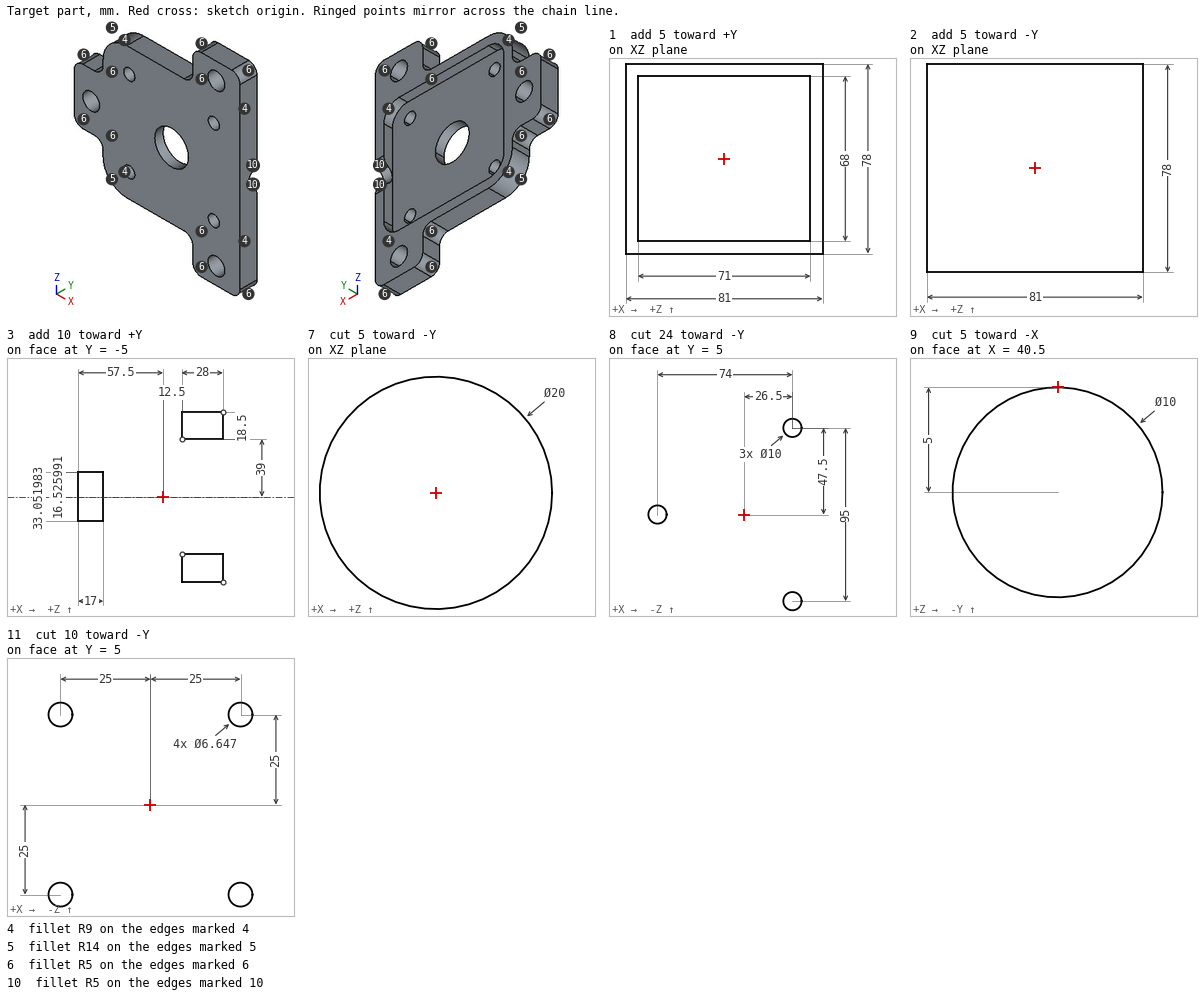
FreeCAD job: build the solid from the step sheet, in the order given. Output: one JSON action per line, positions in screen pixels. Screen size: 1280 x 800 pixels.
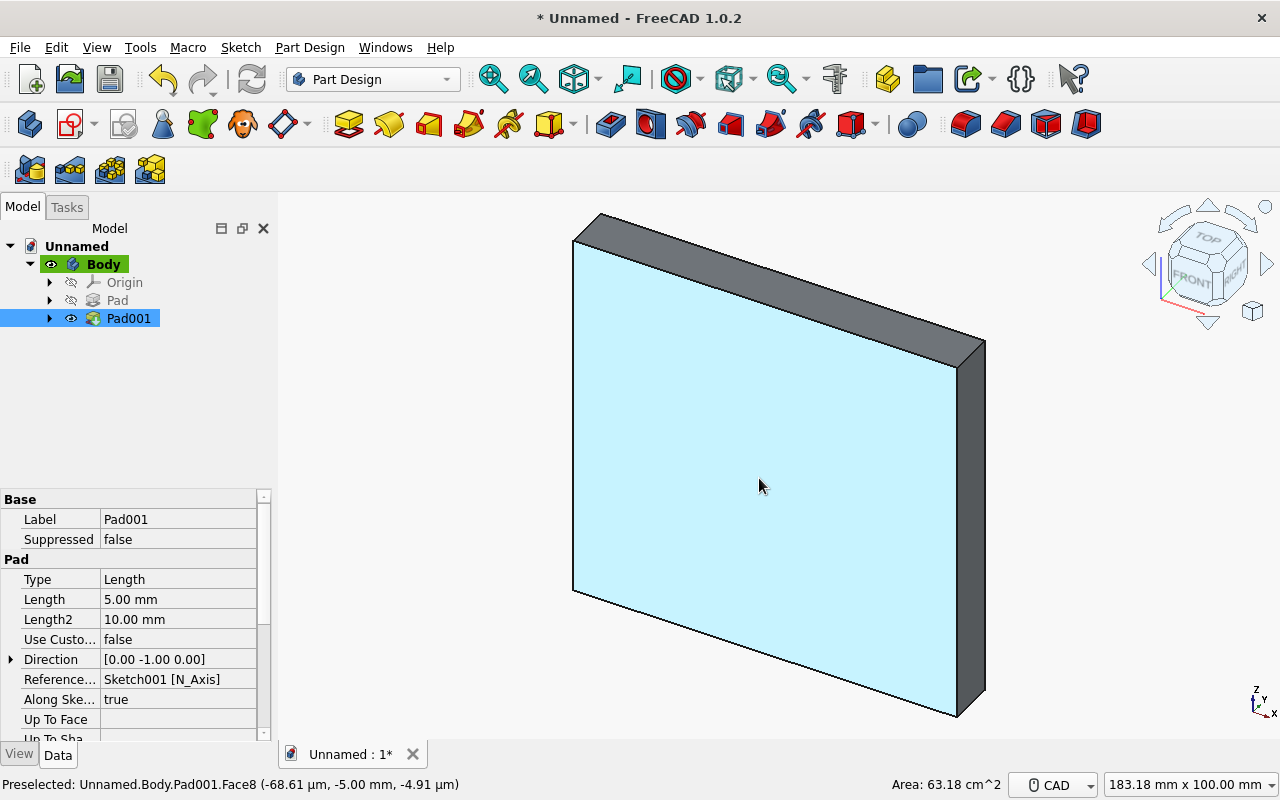
{"action": "left_click", "coordinate": [70, 124]}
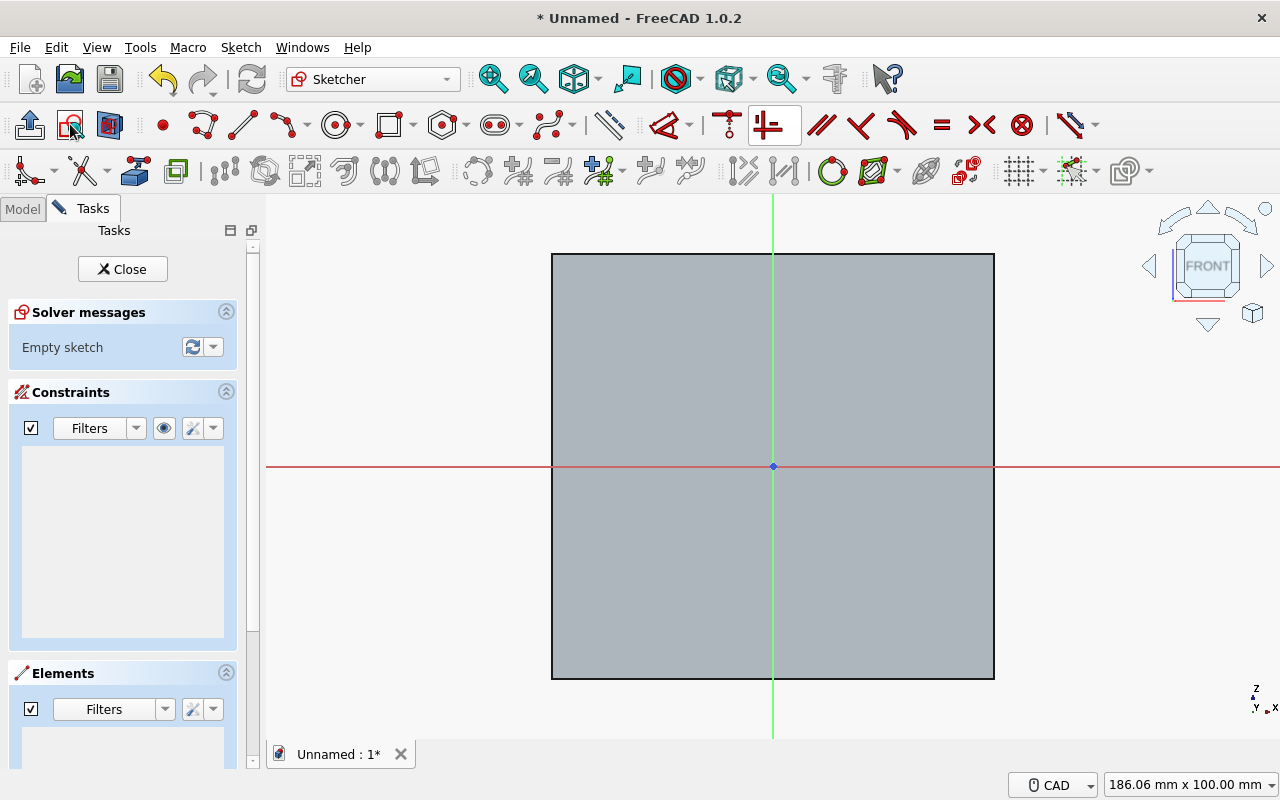
{"action": "scroll", "coordinate": [678, 466], "scroll_direction": "down", "scroll_amount": 3}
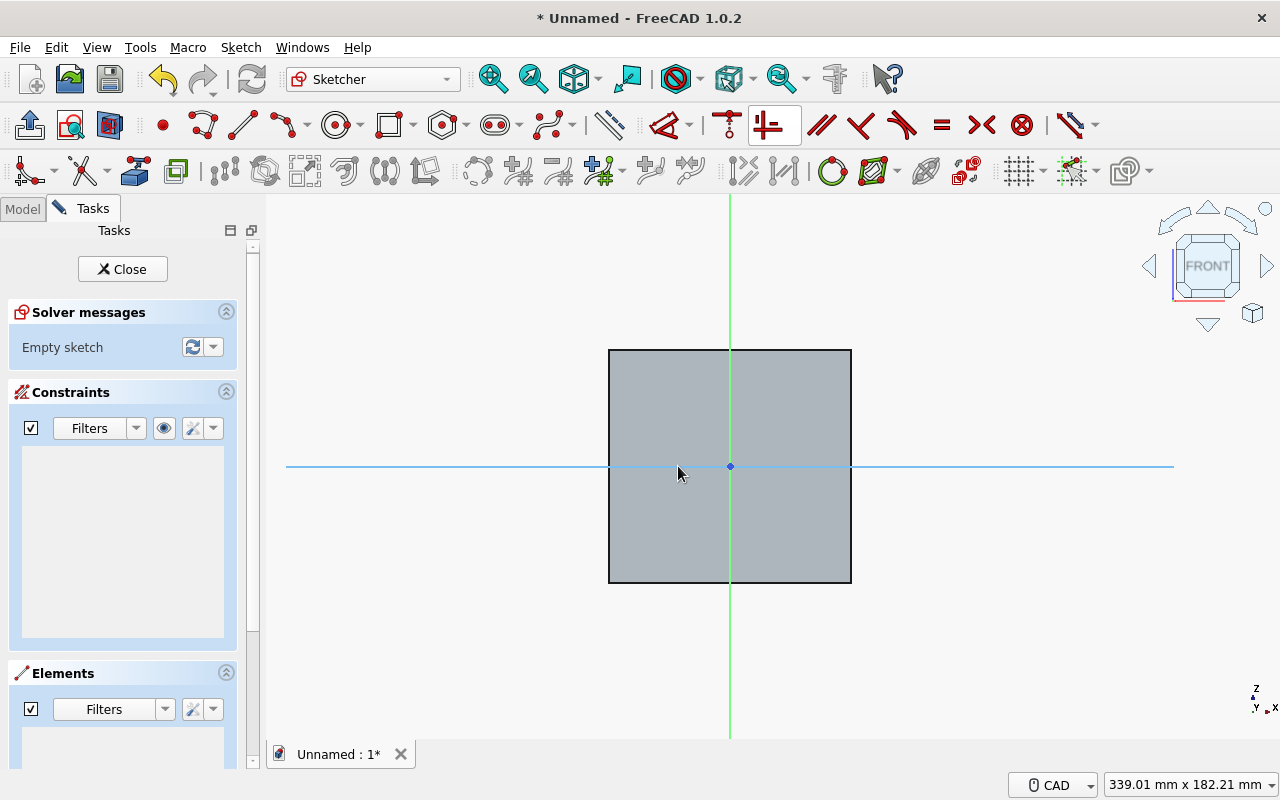
{"action": "left_click", "coordinate": [390, 126]}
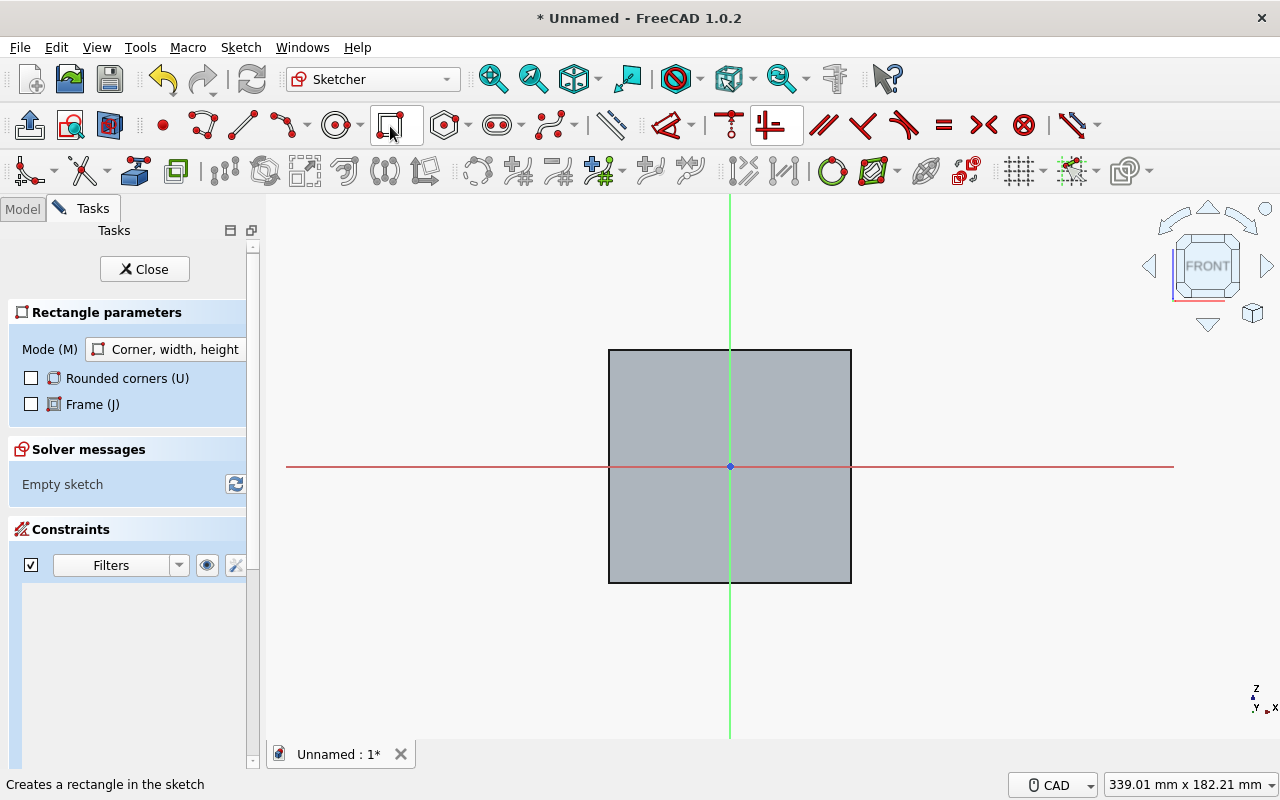
{"action": "left_click", "coordinate": [558, 417]}
{"action": "left_click", "coordinate": [609, 516]}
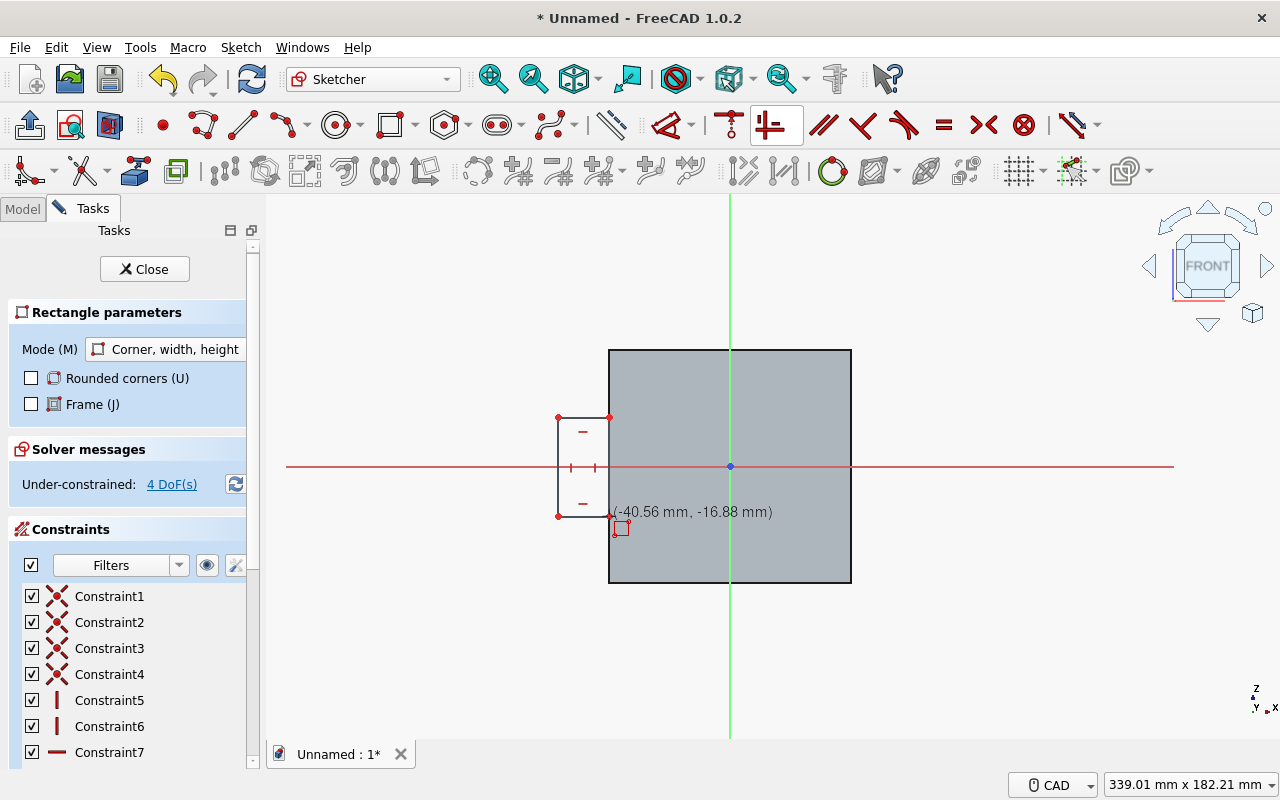
{"action": "left_click", "coordinate": [768, 295]}
{"action": "left_click", "coordinate": [851, 350]}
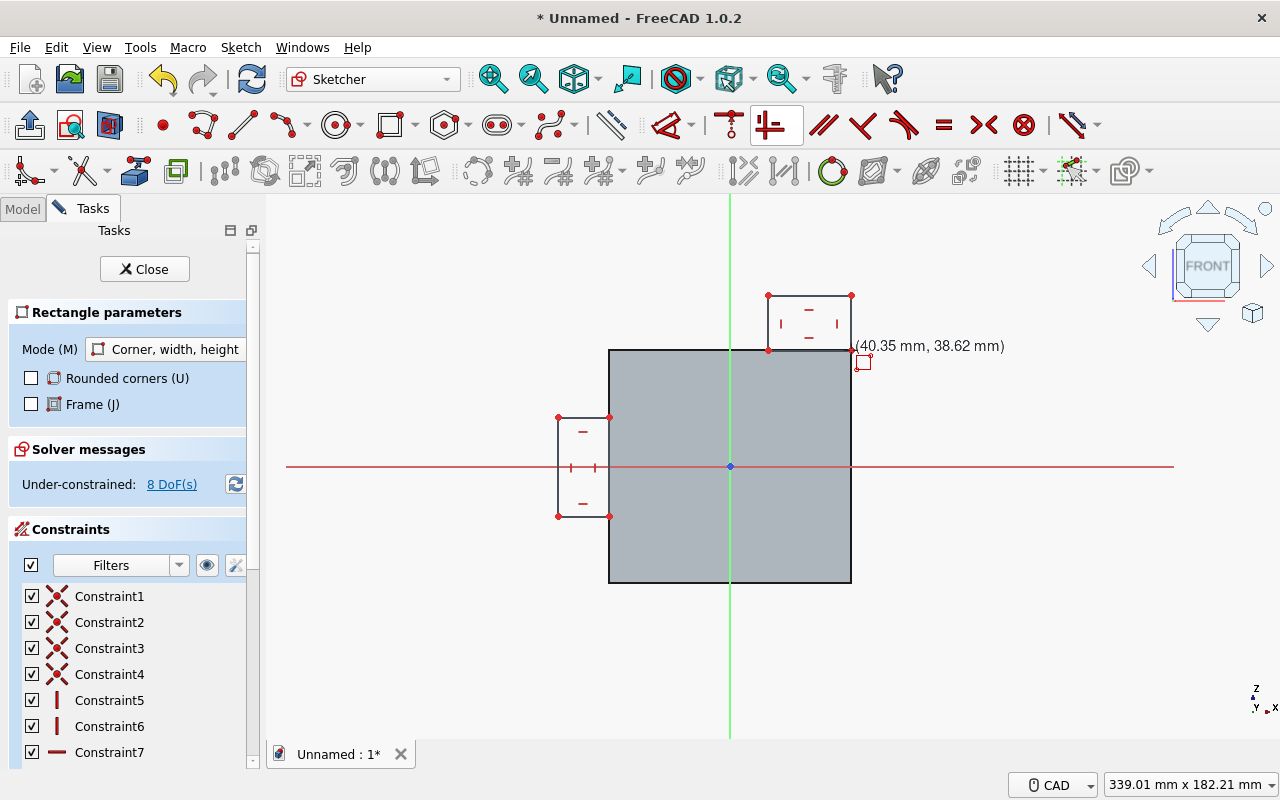
{"action": "left_click", "coordinate": [768, 583]}
{"action": "left_click", "coordinate": [851, 638]}
{"action": "key", "text": "Escape"}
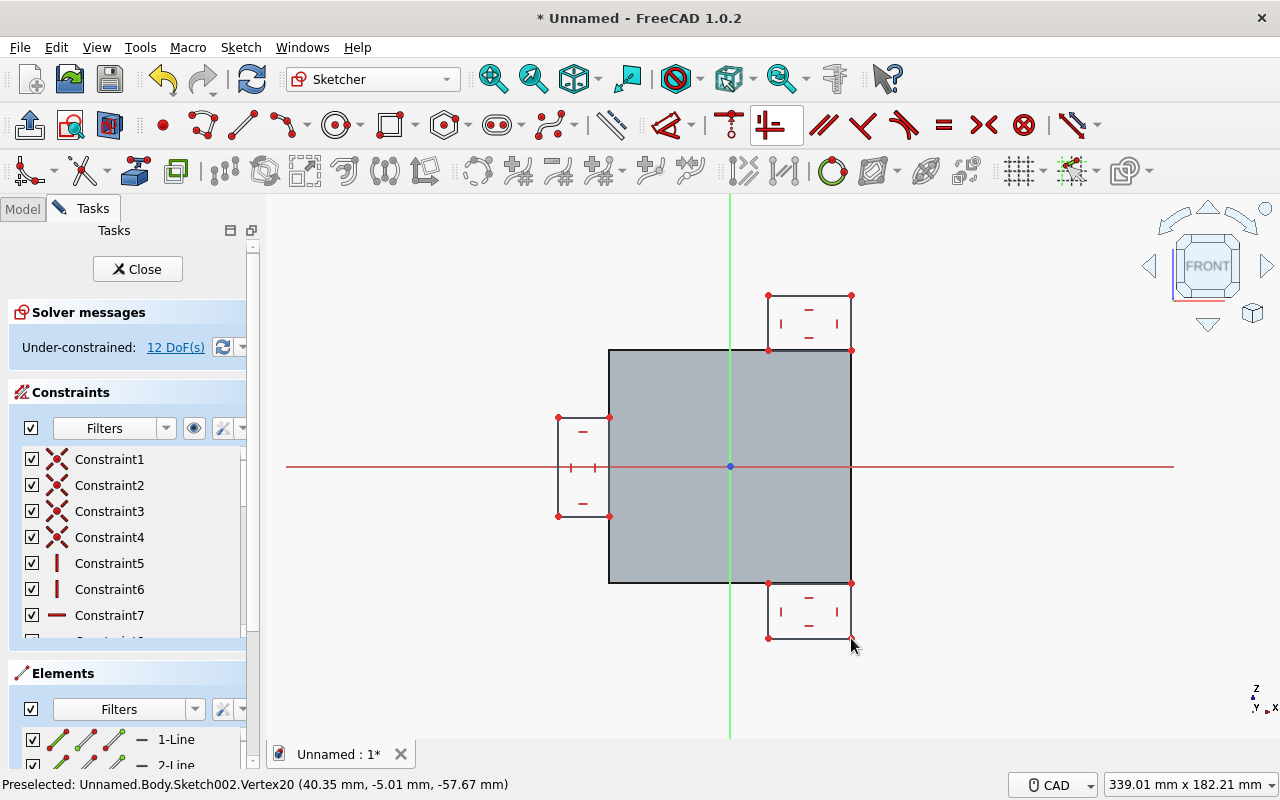
{"action": "left_click", "coordinate": [768, 351]}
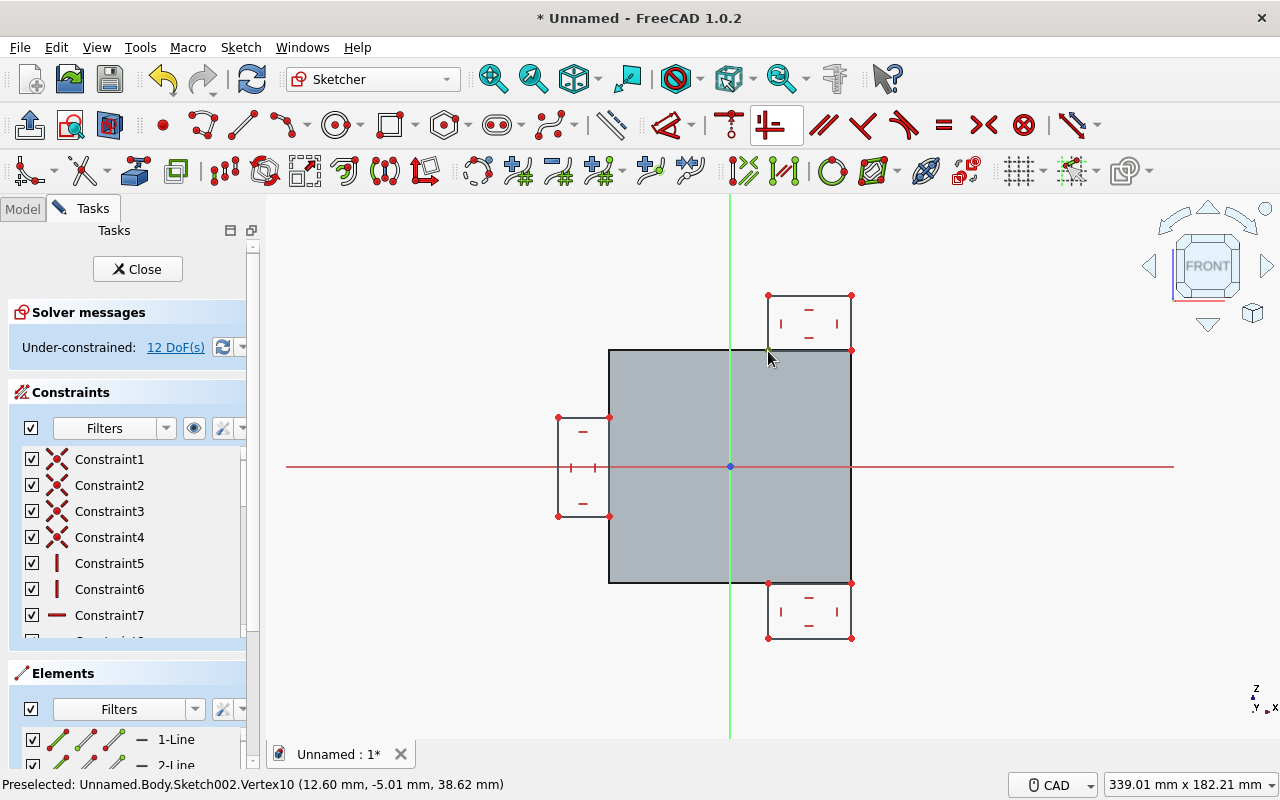
{"action": "left_click", "coordinate": [768, 584]}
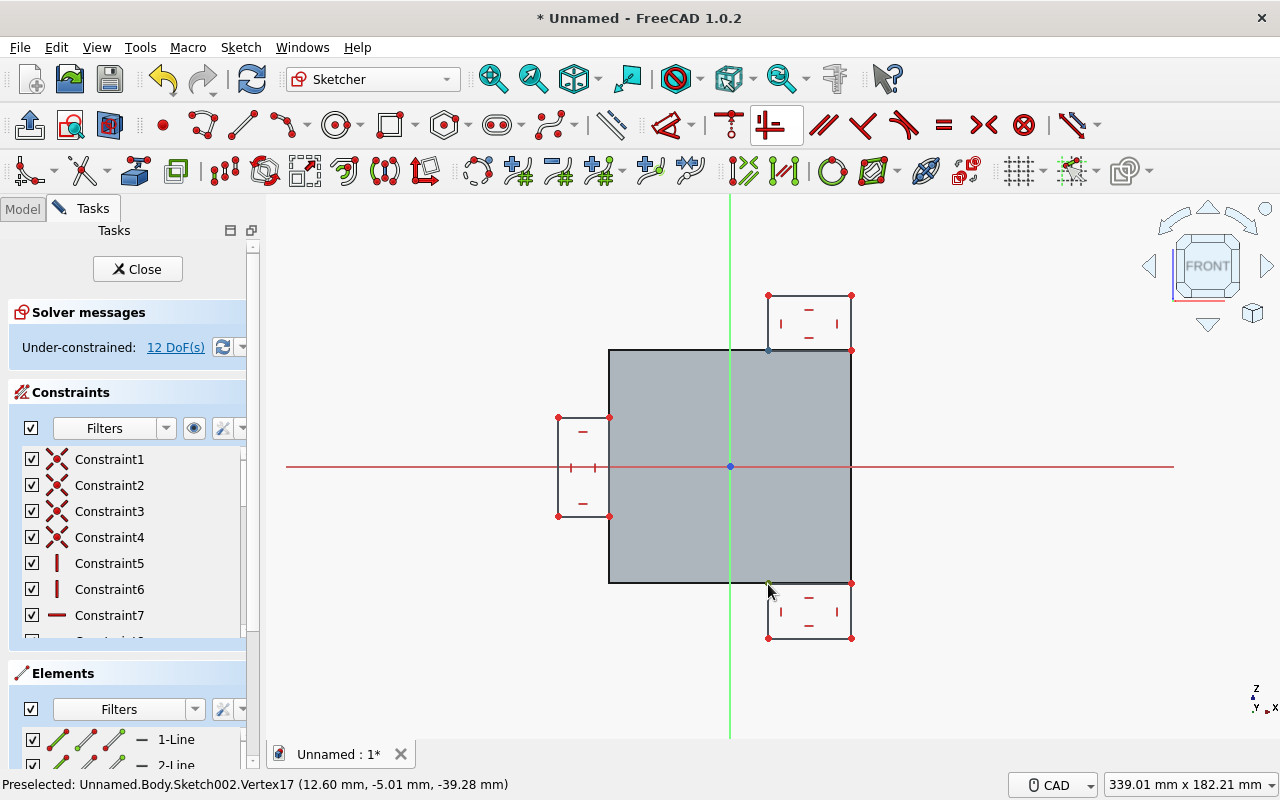
{"action": "left_click", "coordinate": [353, 466]}